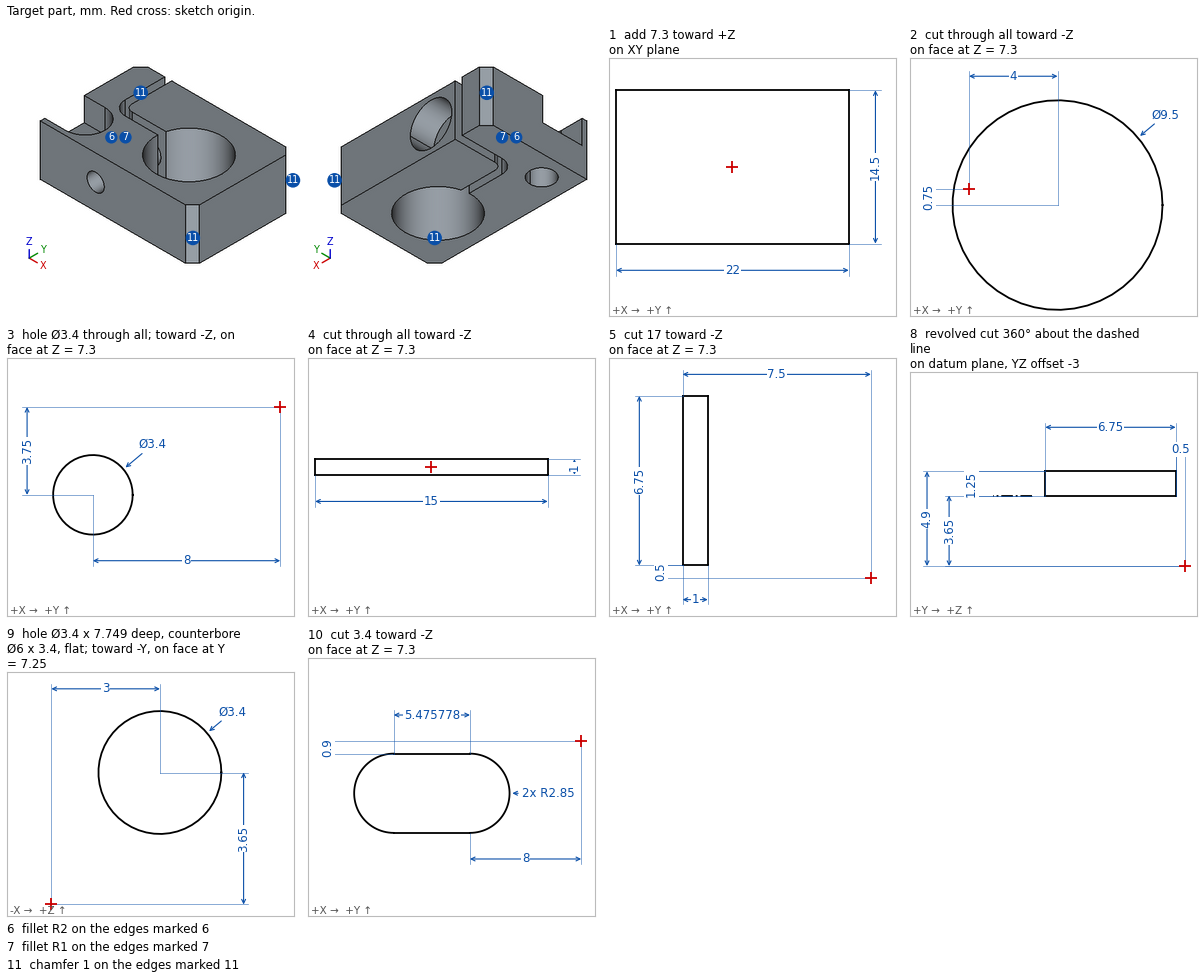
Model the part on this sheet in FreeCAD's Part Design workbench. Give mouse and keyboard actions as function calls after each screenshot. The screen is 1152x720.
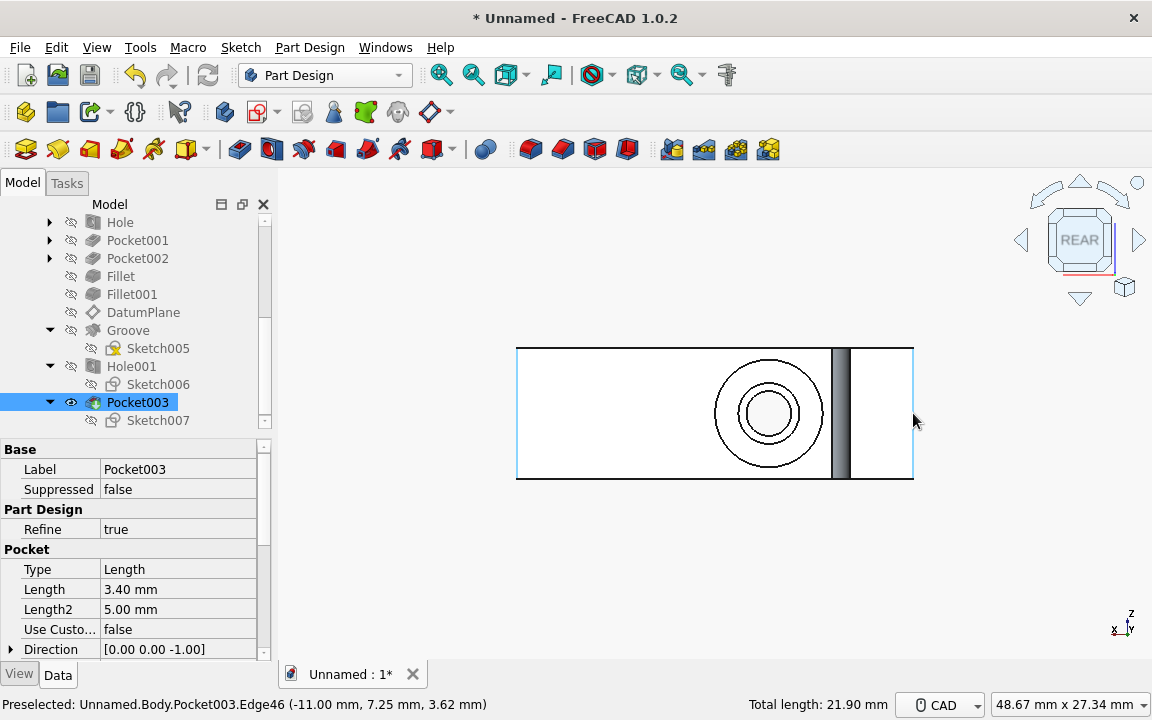
click(564, 150)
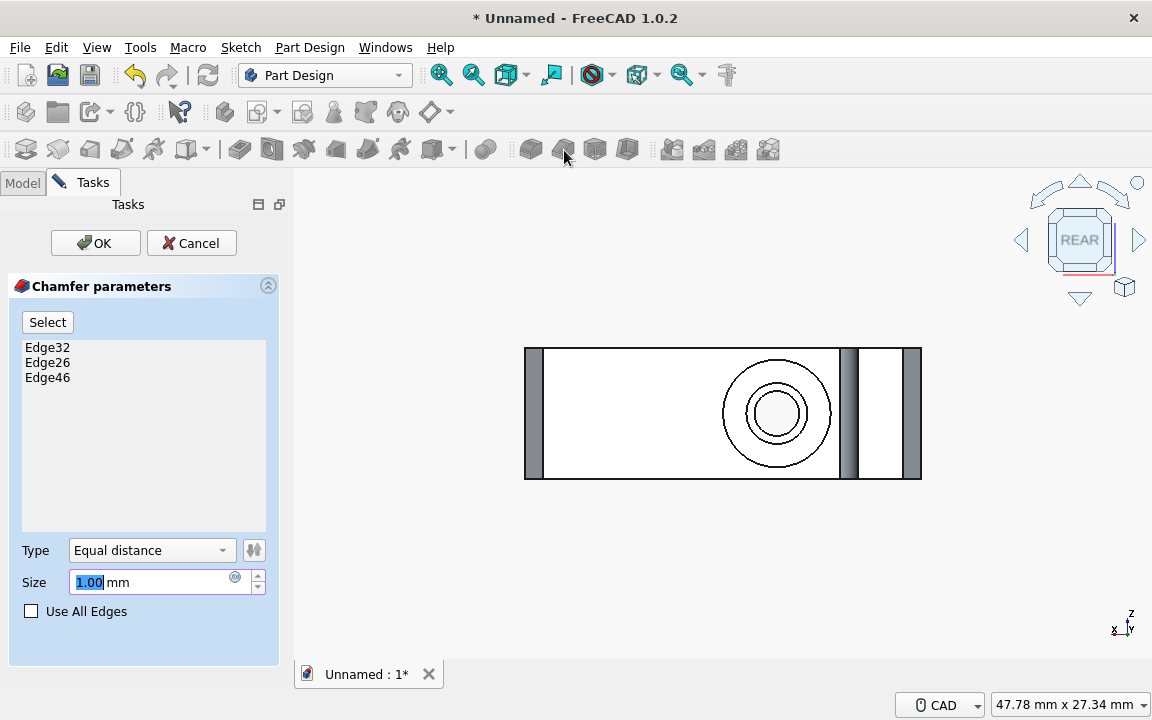
text(1)
key(Tab)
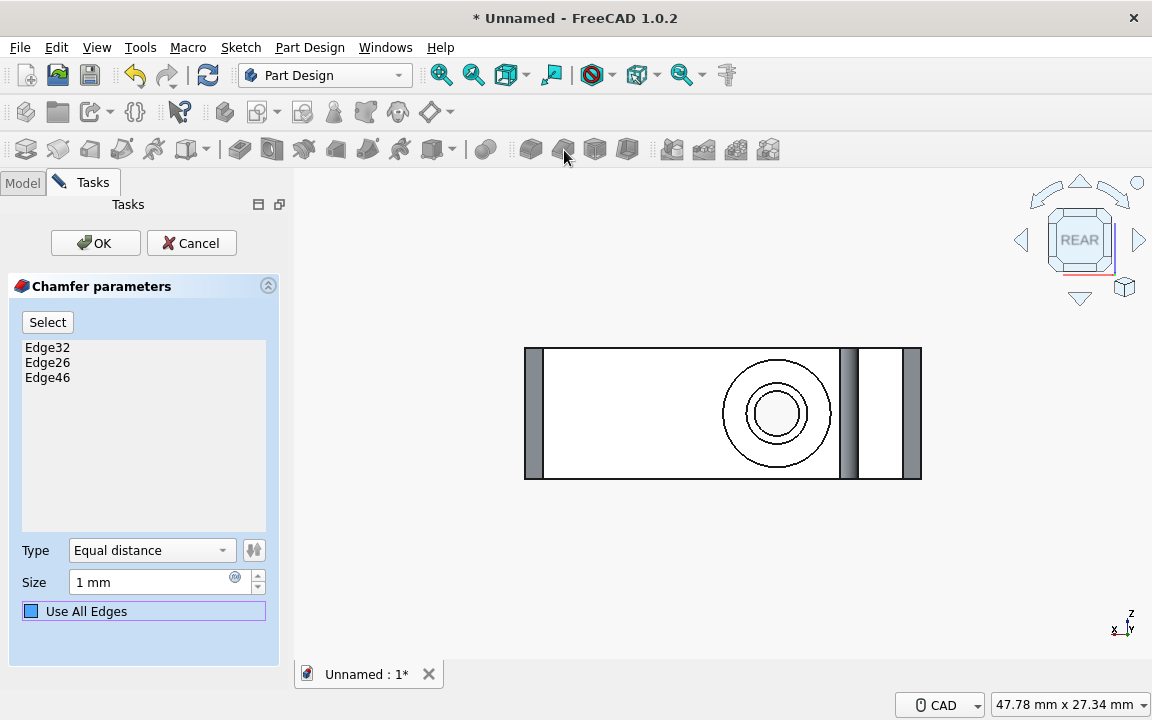
click(96, 243)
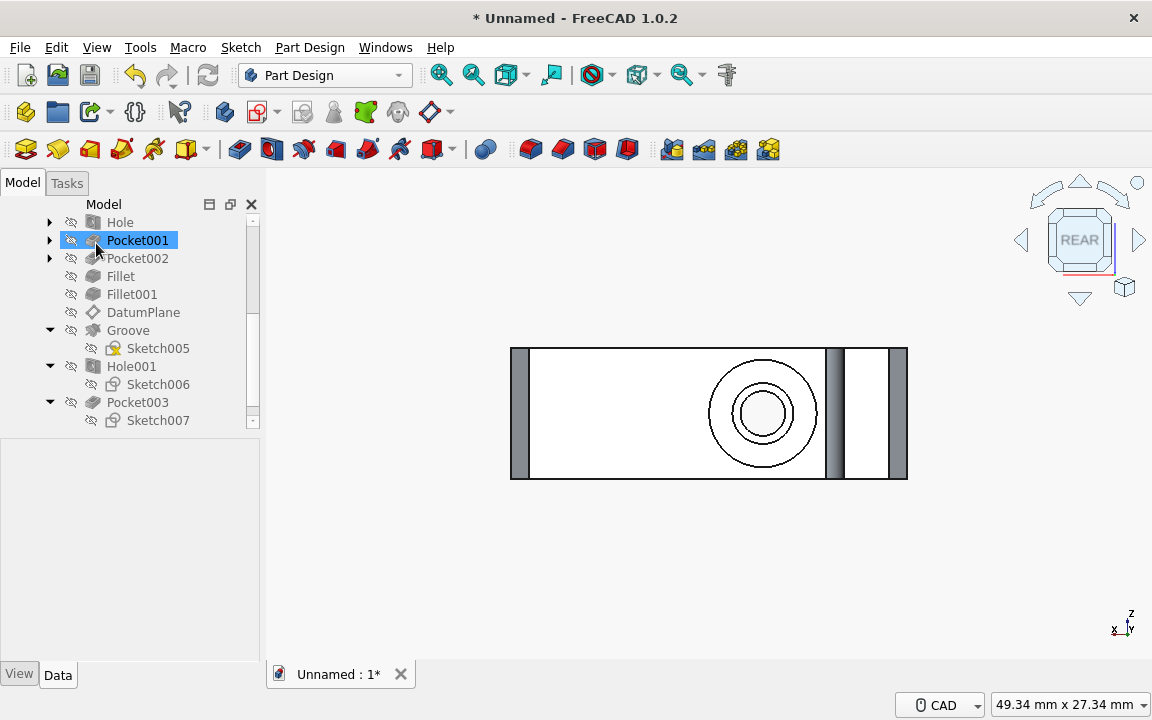
key(0)